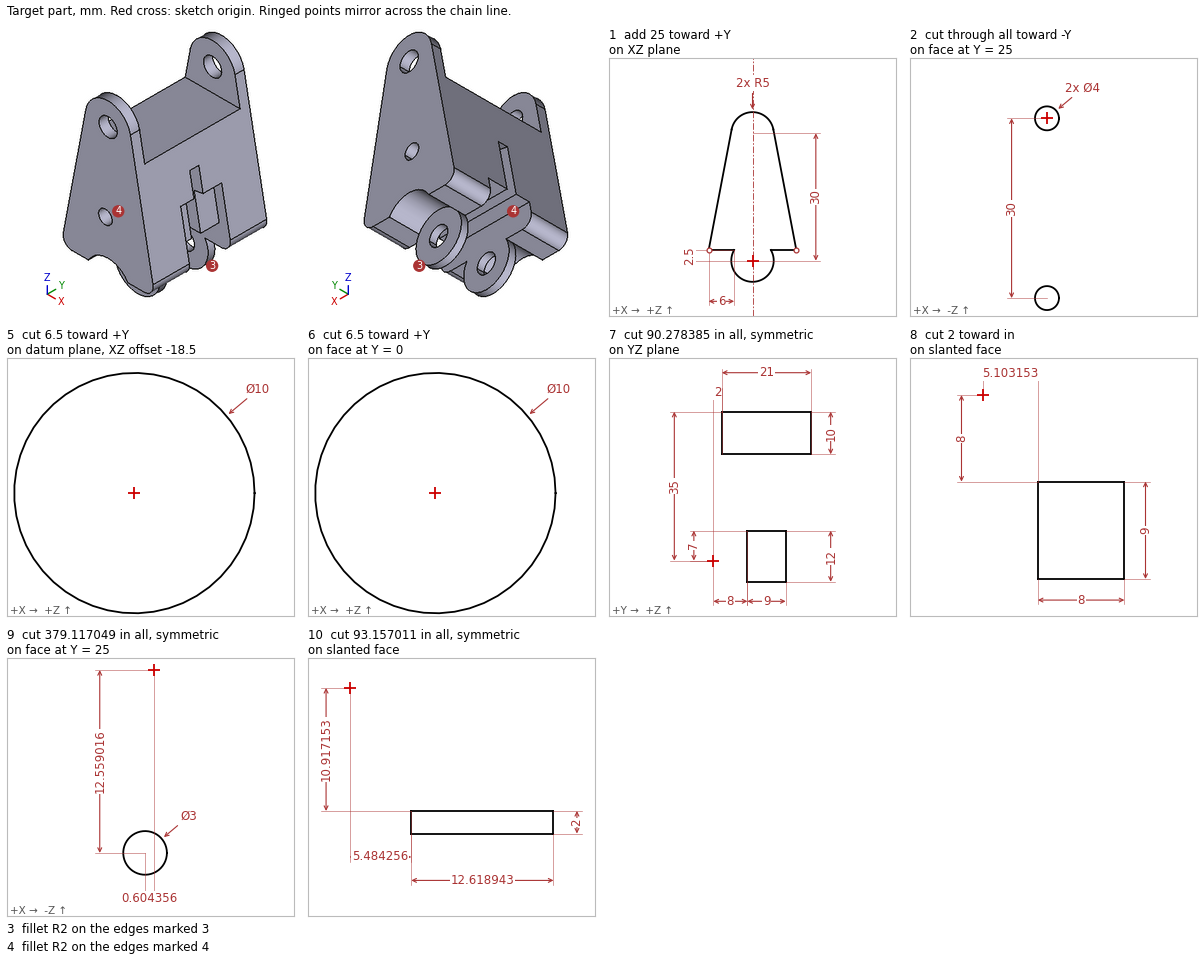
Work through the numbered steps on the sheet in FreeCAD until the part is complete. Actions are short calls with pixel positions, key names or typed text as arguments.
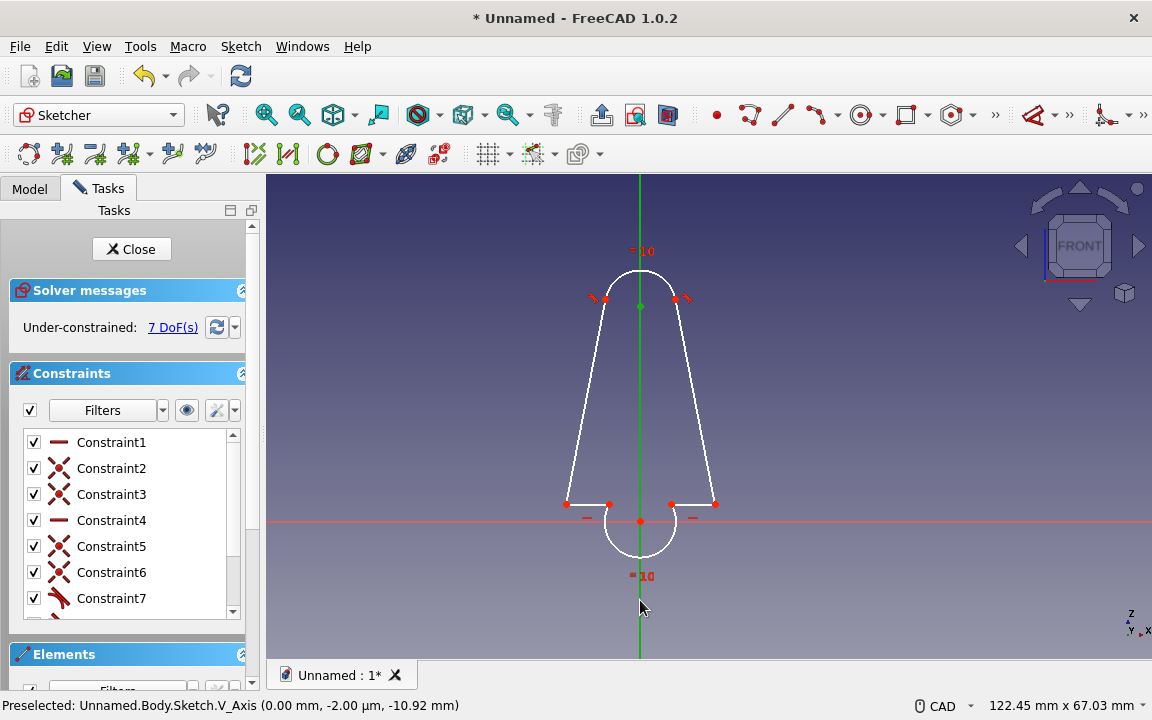
key(c)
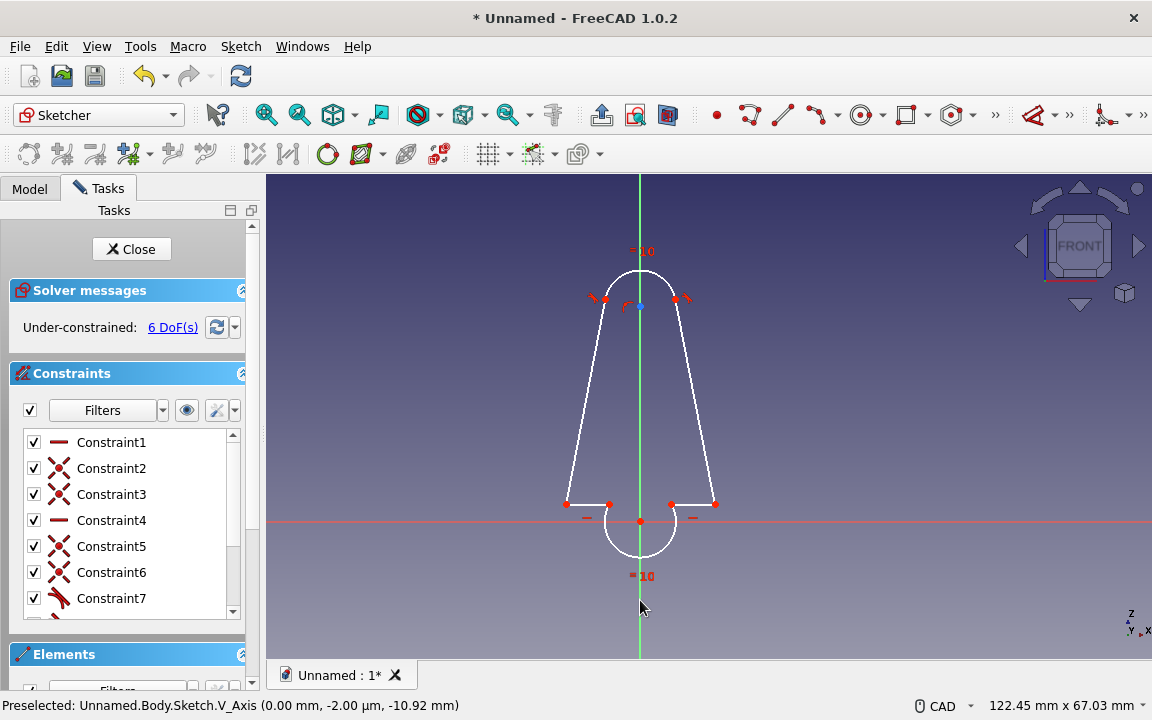
click(566, 505)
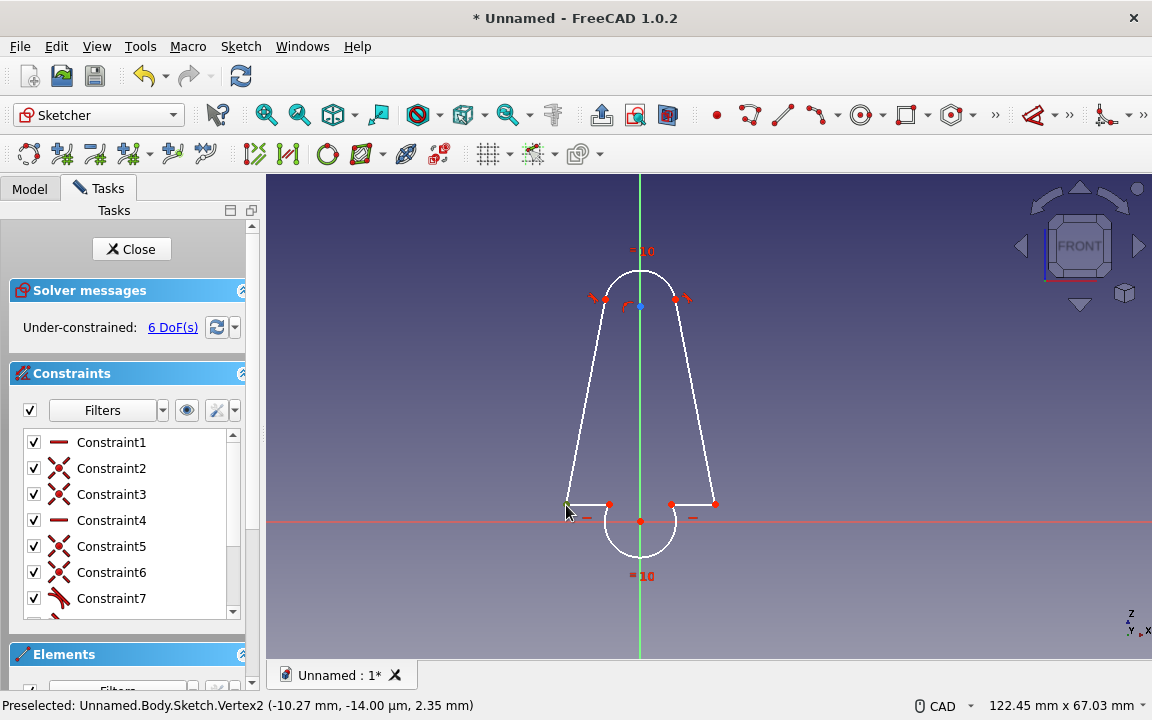
click(715, 505)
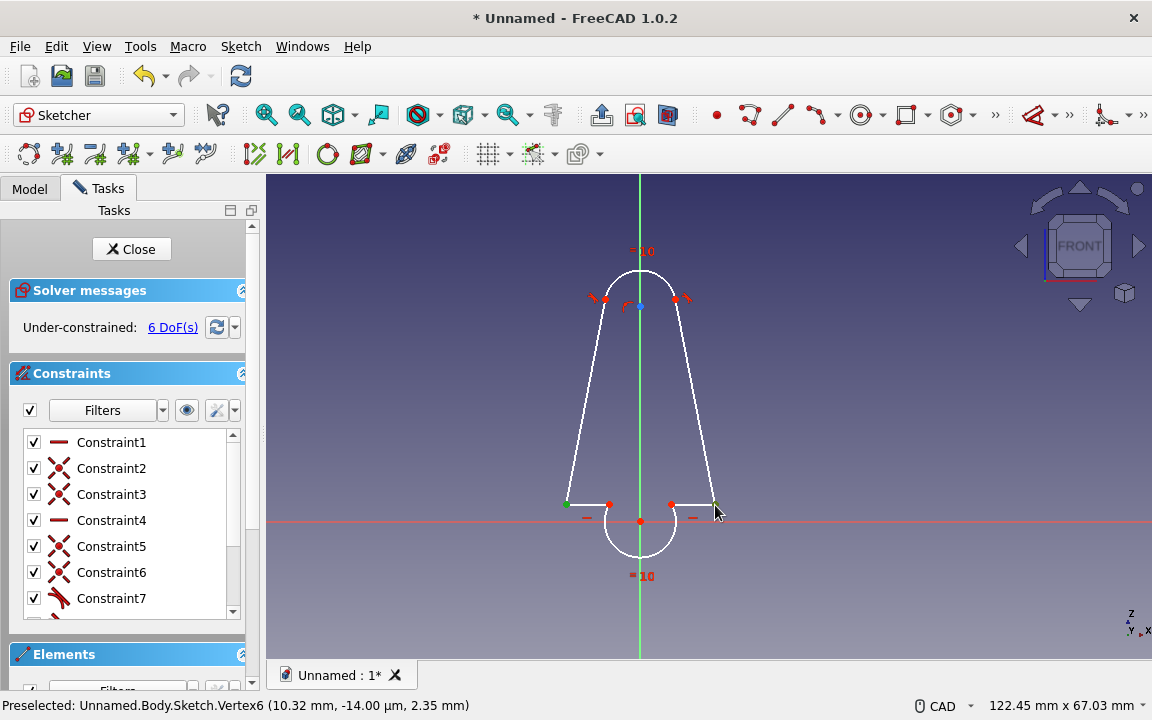
click(640, 600)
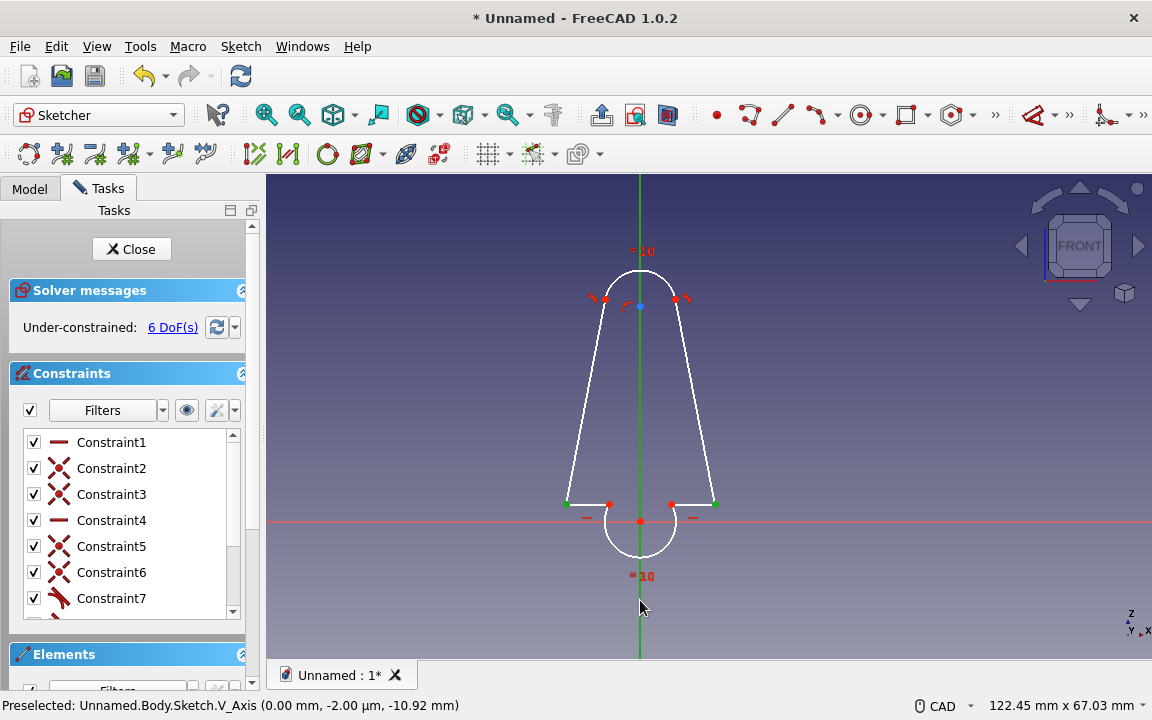
key(s)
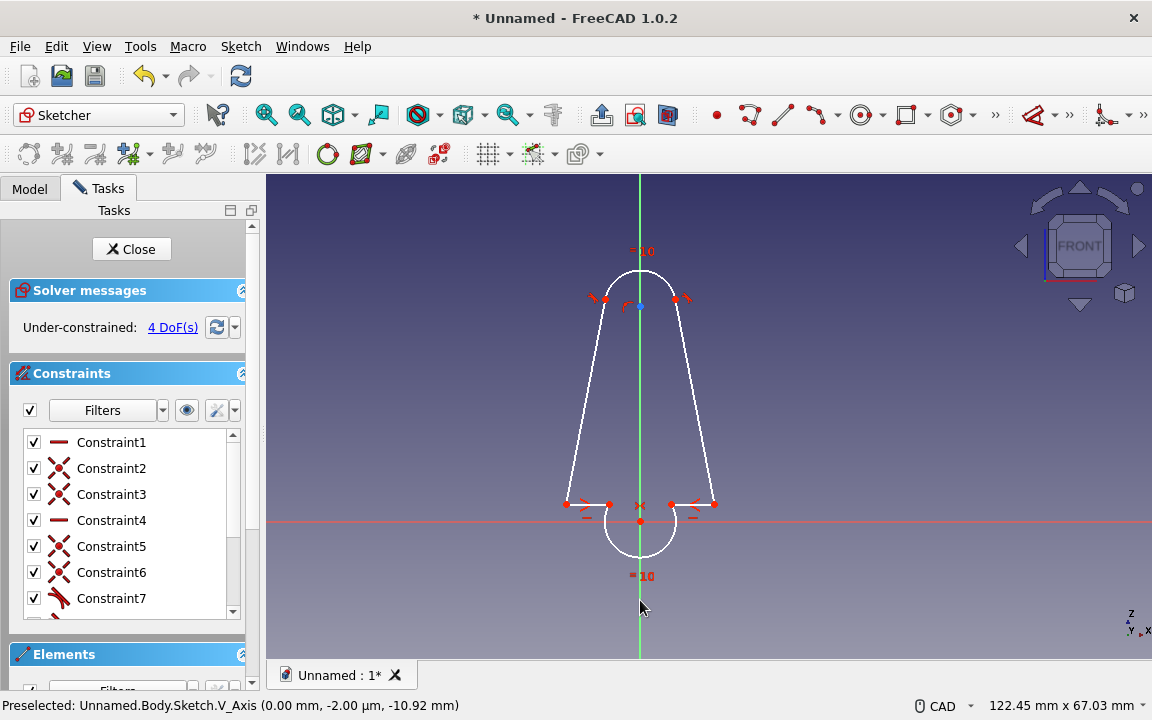
key(d)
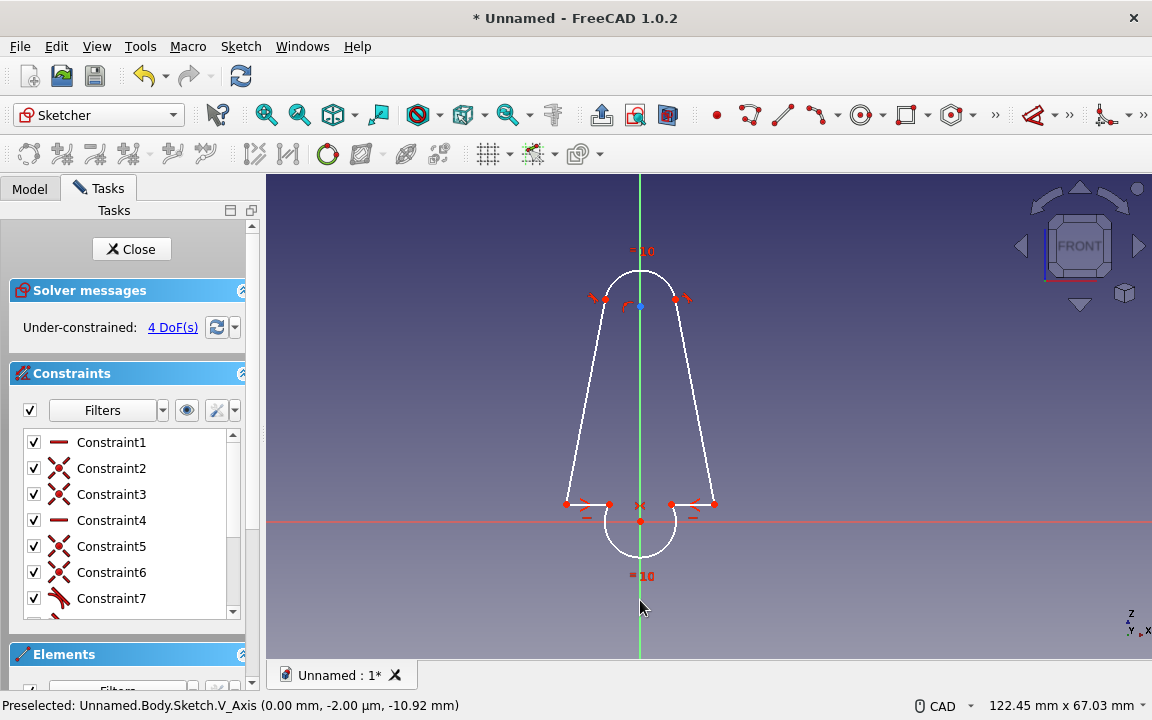
click(659, 276)
click(676, 249)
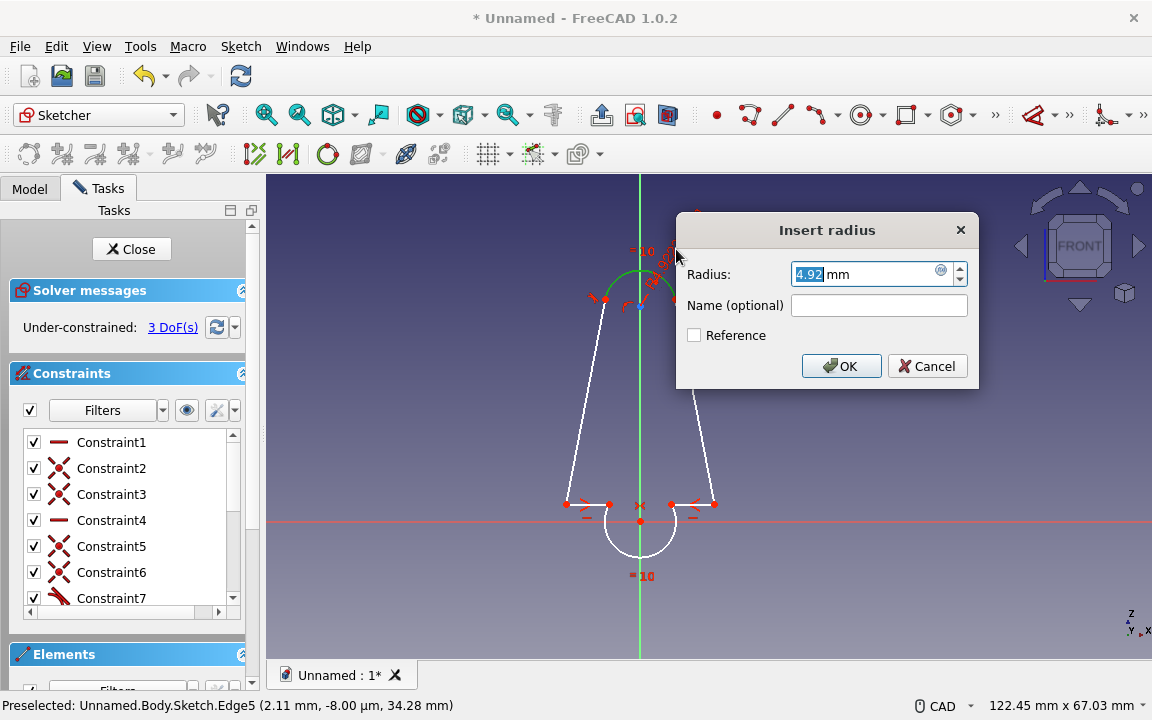
text(5)
key(Return)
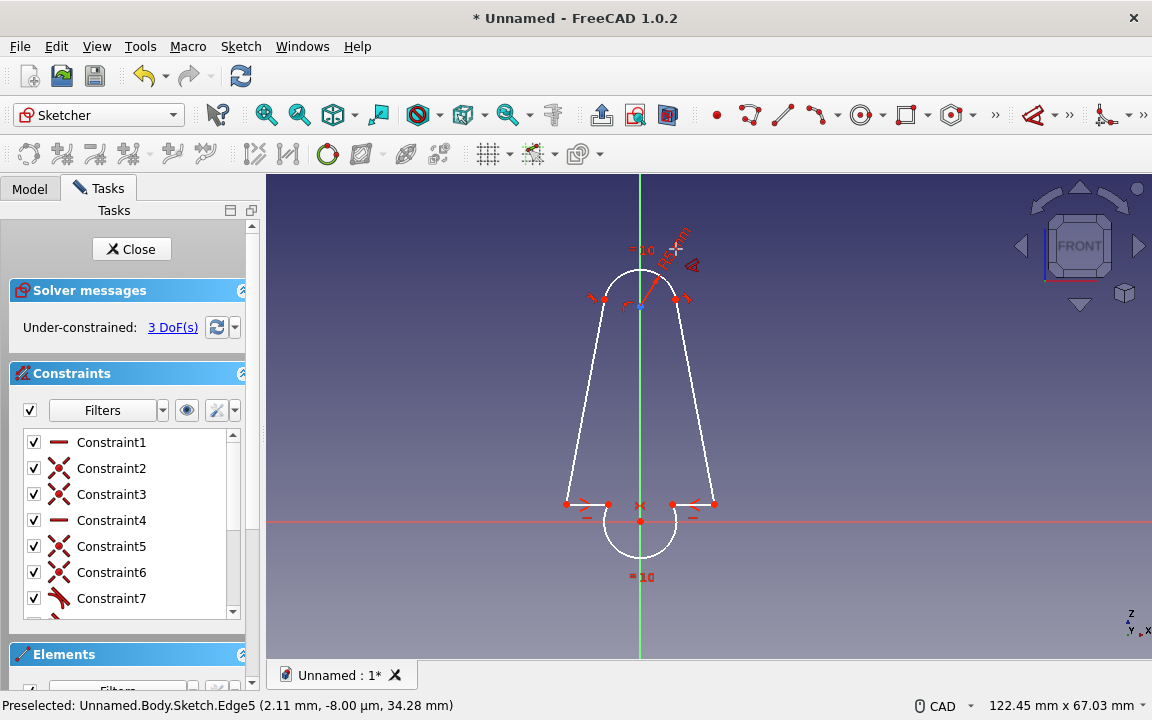
click(596, 505)
click(587, 539)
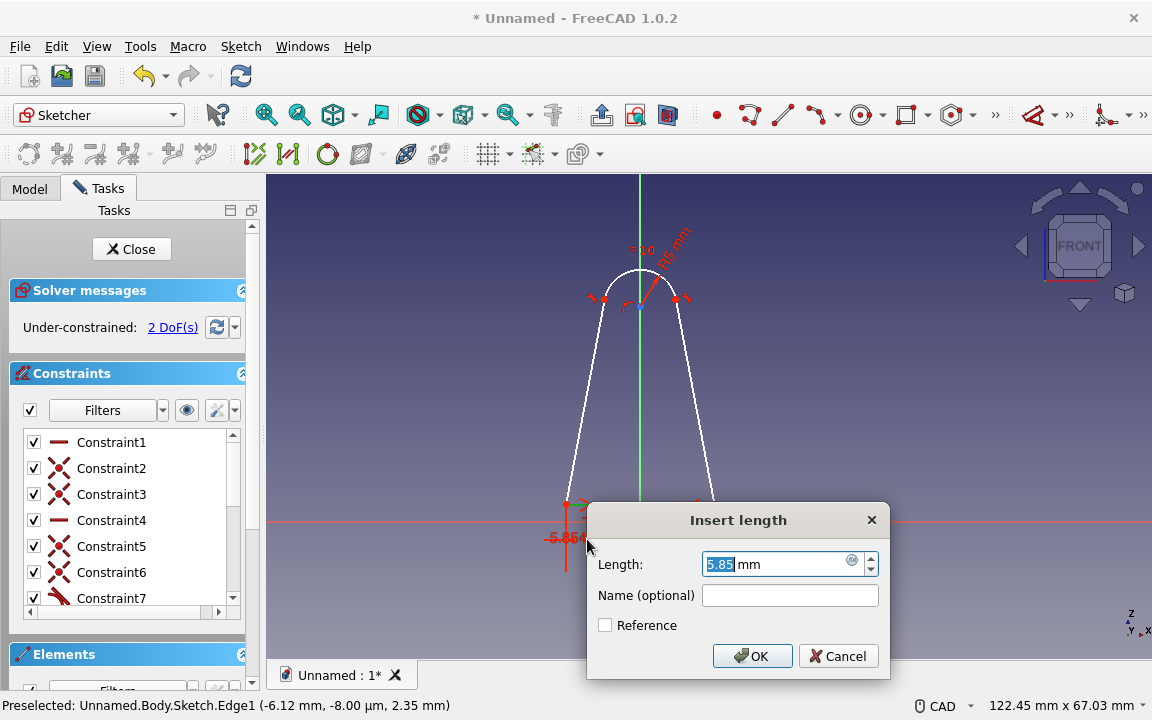
text(6)
key(Return)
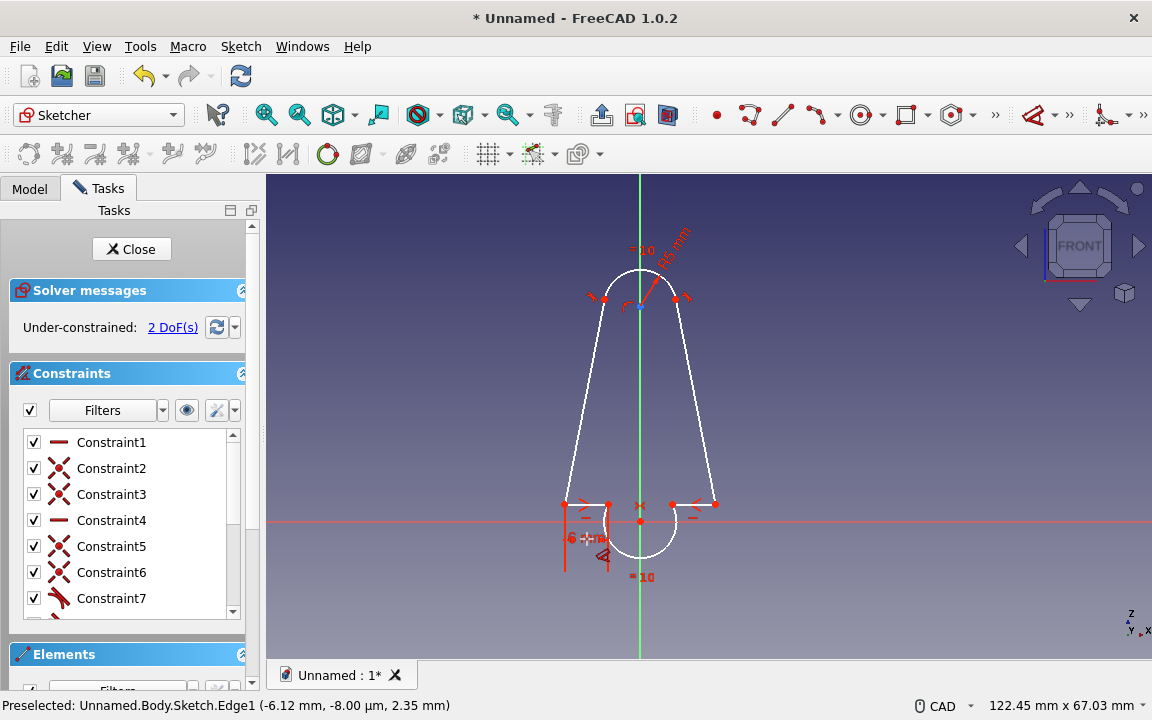
click(640, 306)
click(674, 414)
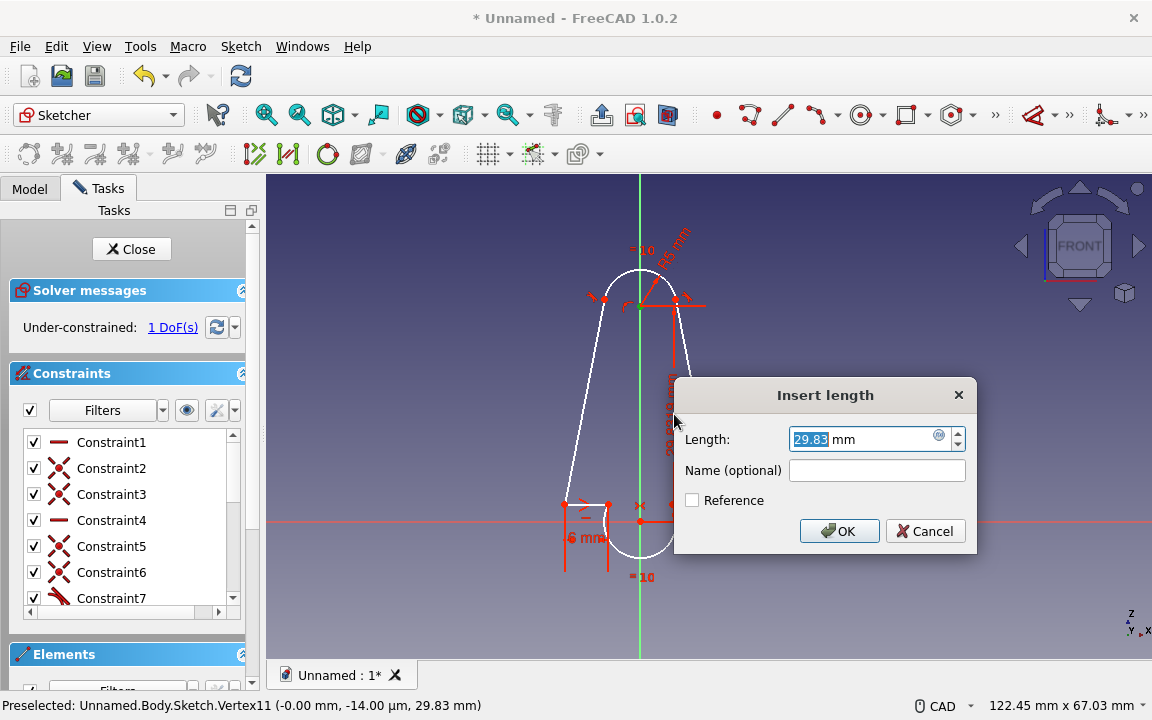
text(30)
key(Return)